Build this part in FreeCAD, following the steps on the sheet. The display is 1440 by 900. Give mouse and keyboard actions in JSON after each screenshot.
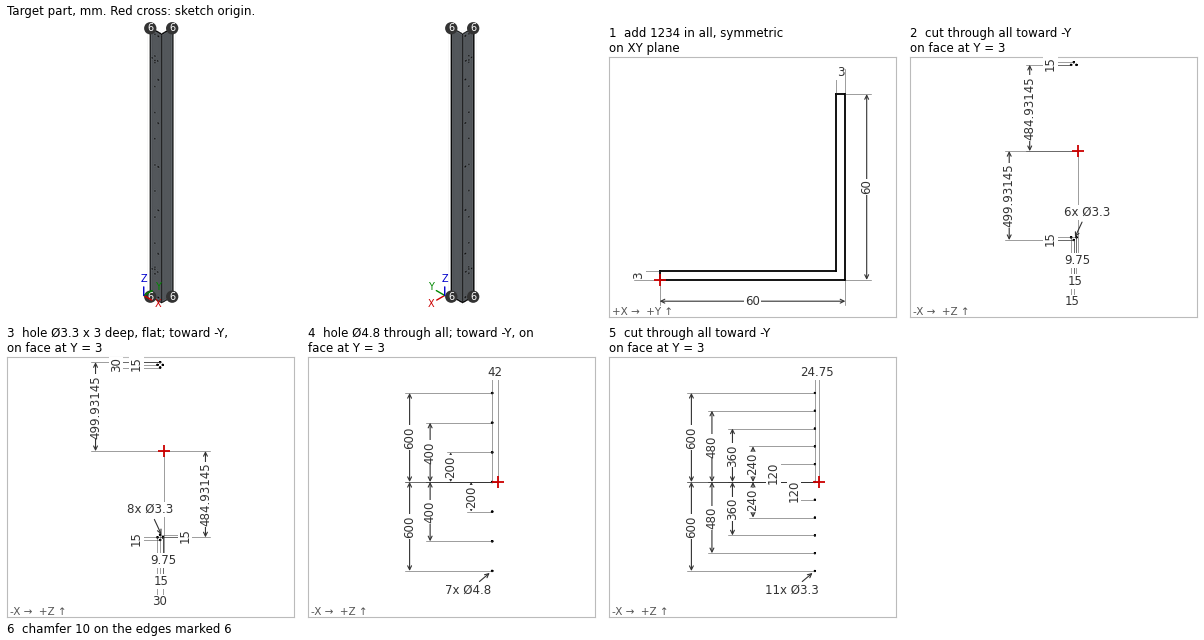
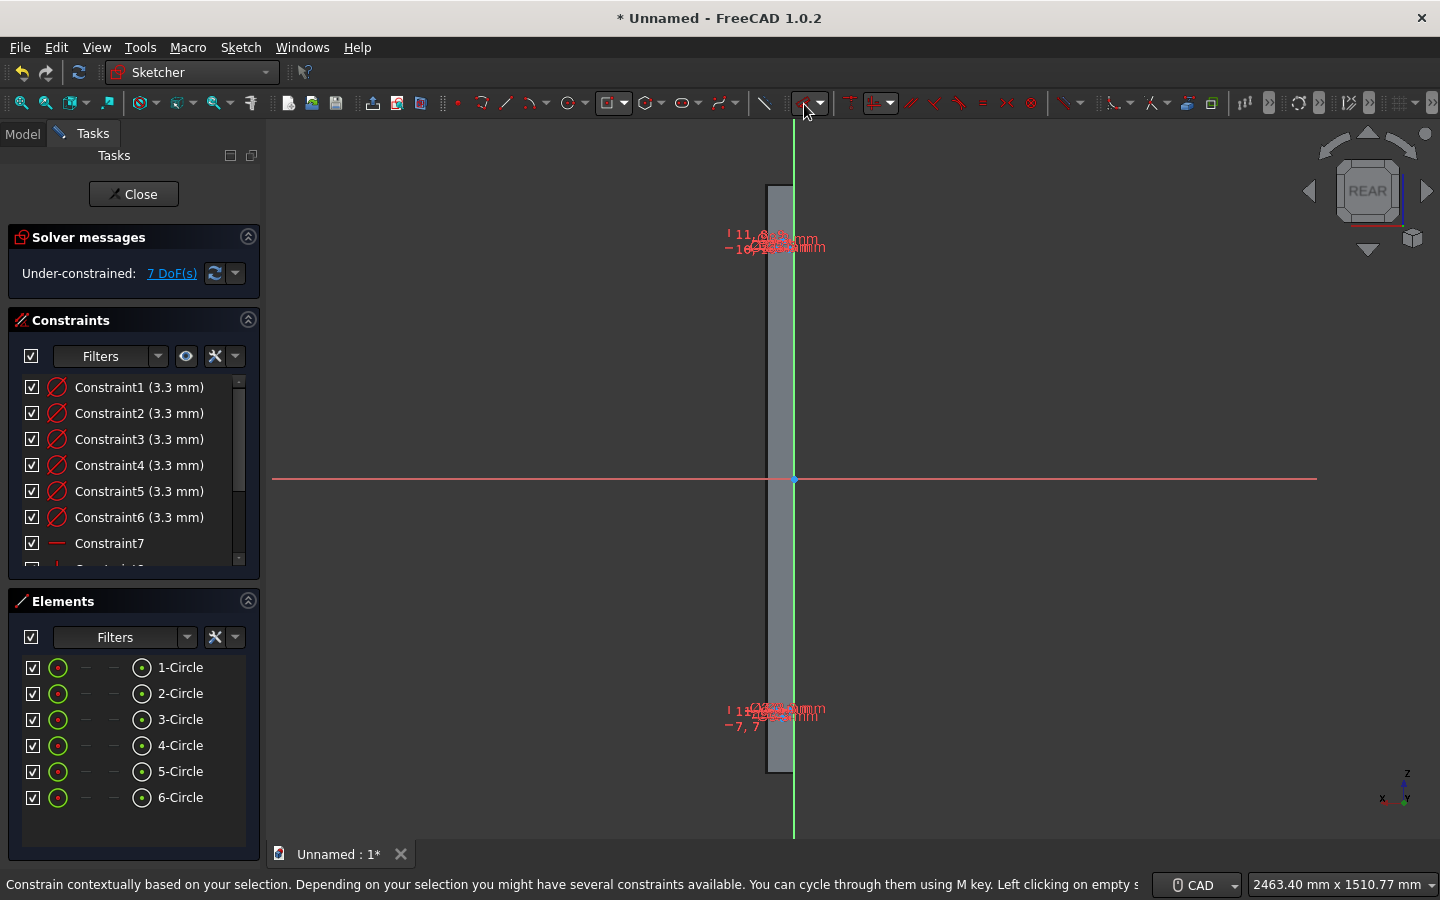
{"action": "scroll", "coordinate": [782, 718], "scroll_direction": "up", "scroll_amount": 9}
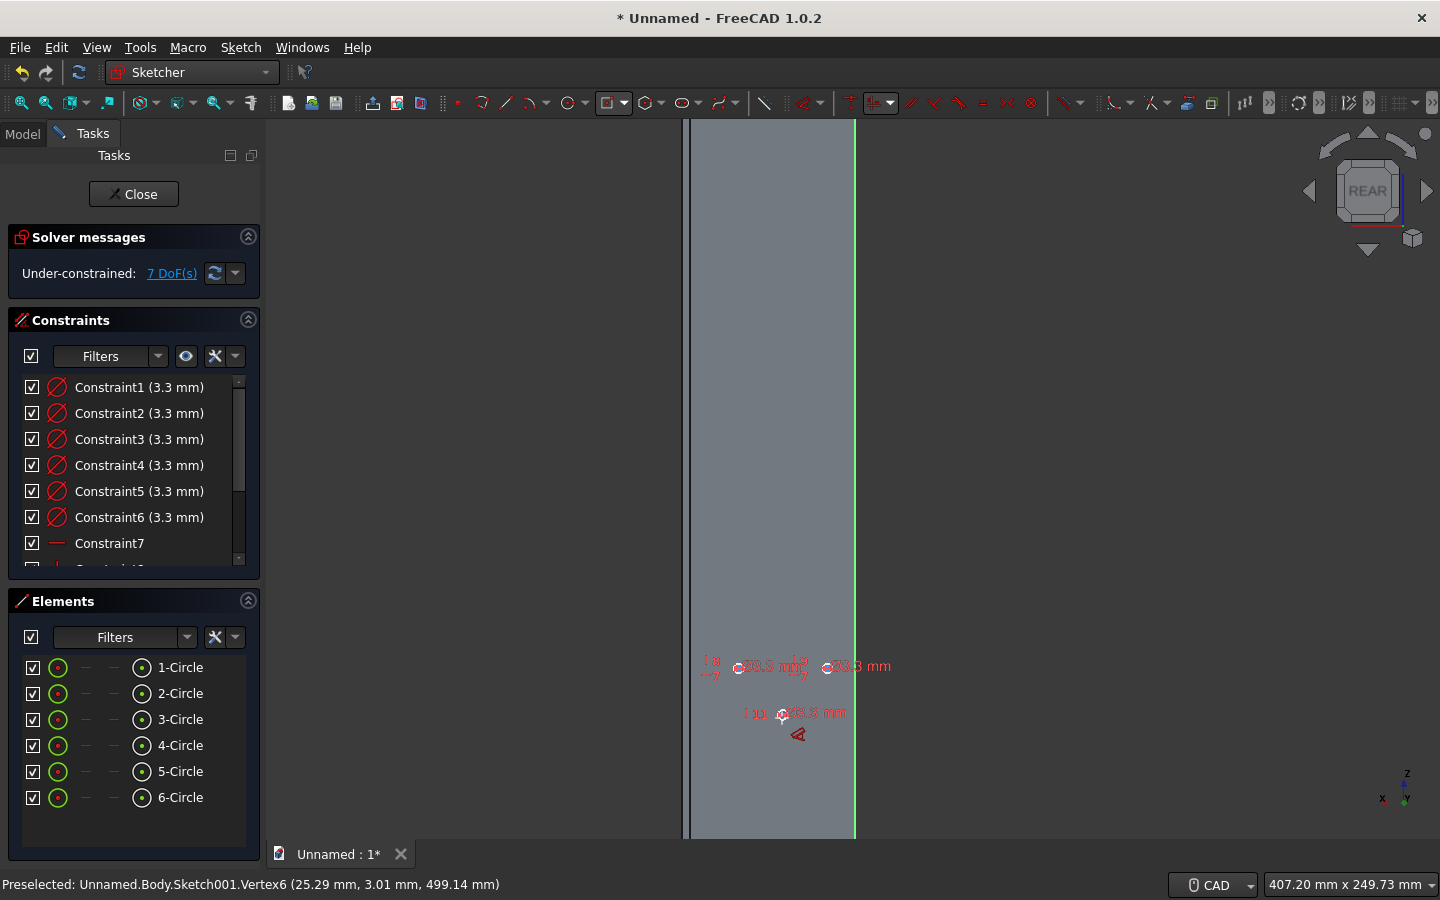
{"action": "left_click", "coordinate": [783, 715]}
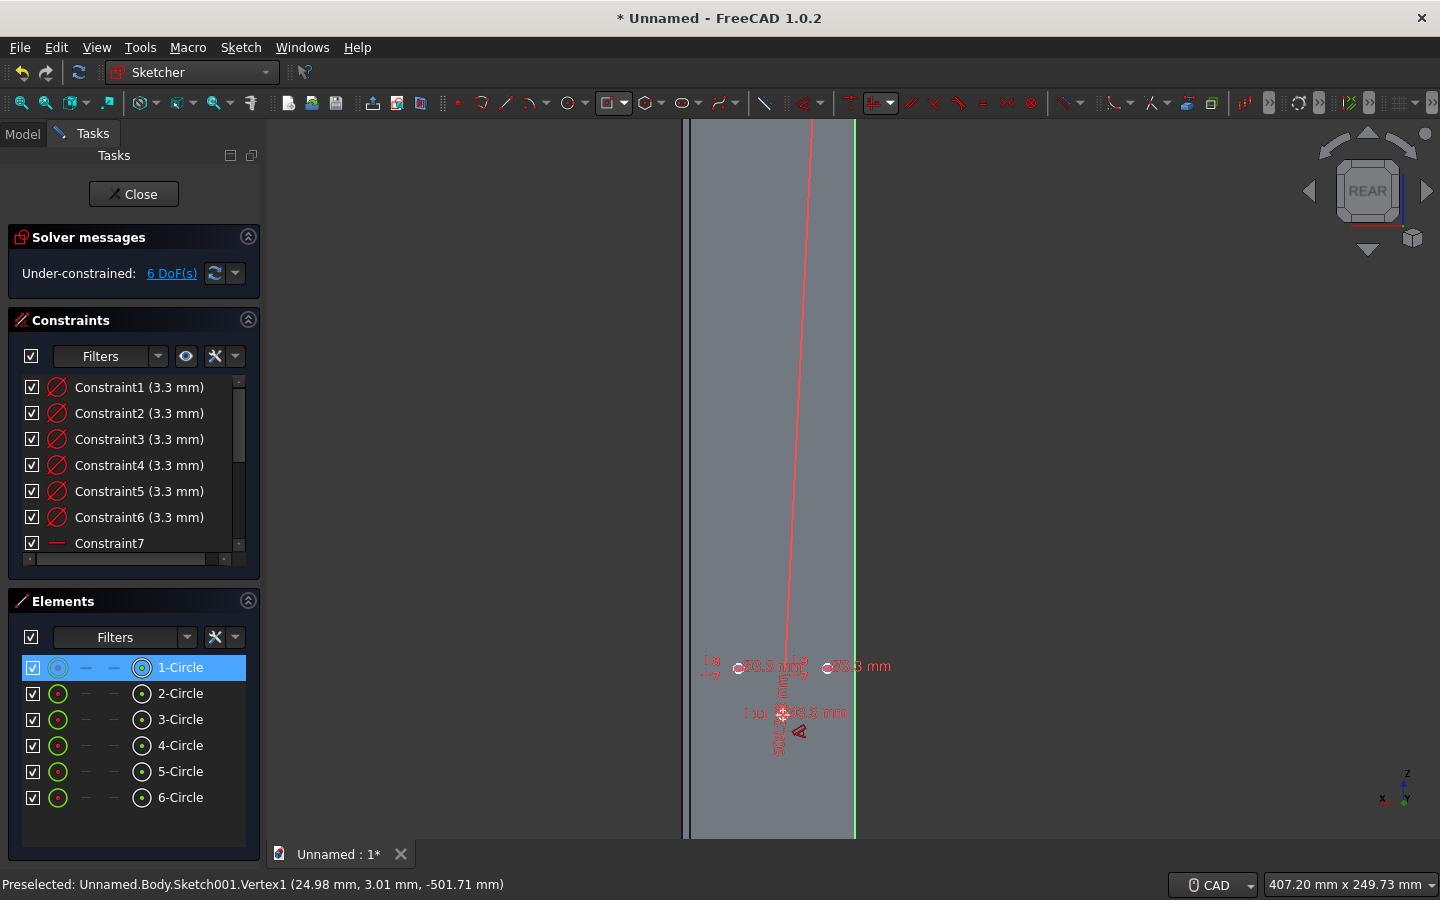
{"action": "left_click", "coordinate": [827, 668]}
{"action": "left_click", "coordinate": [805, 749]}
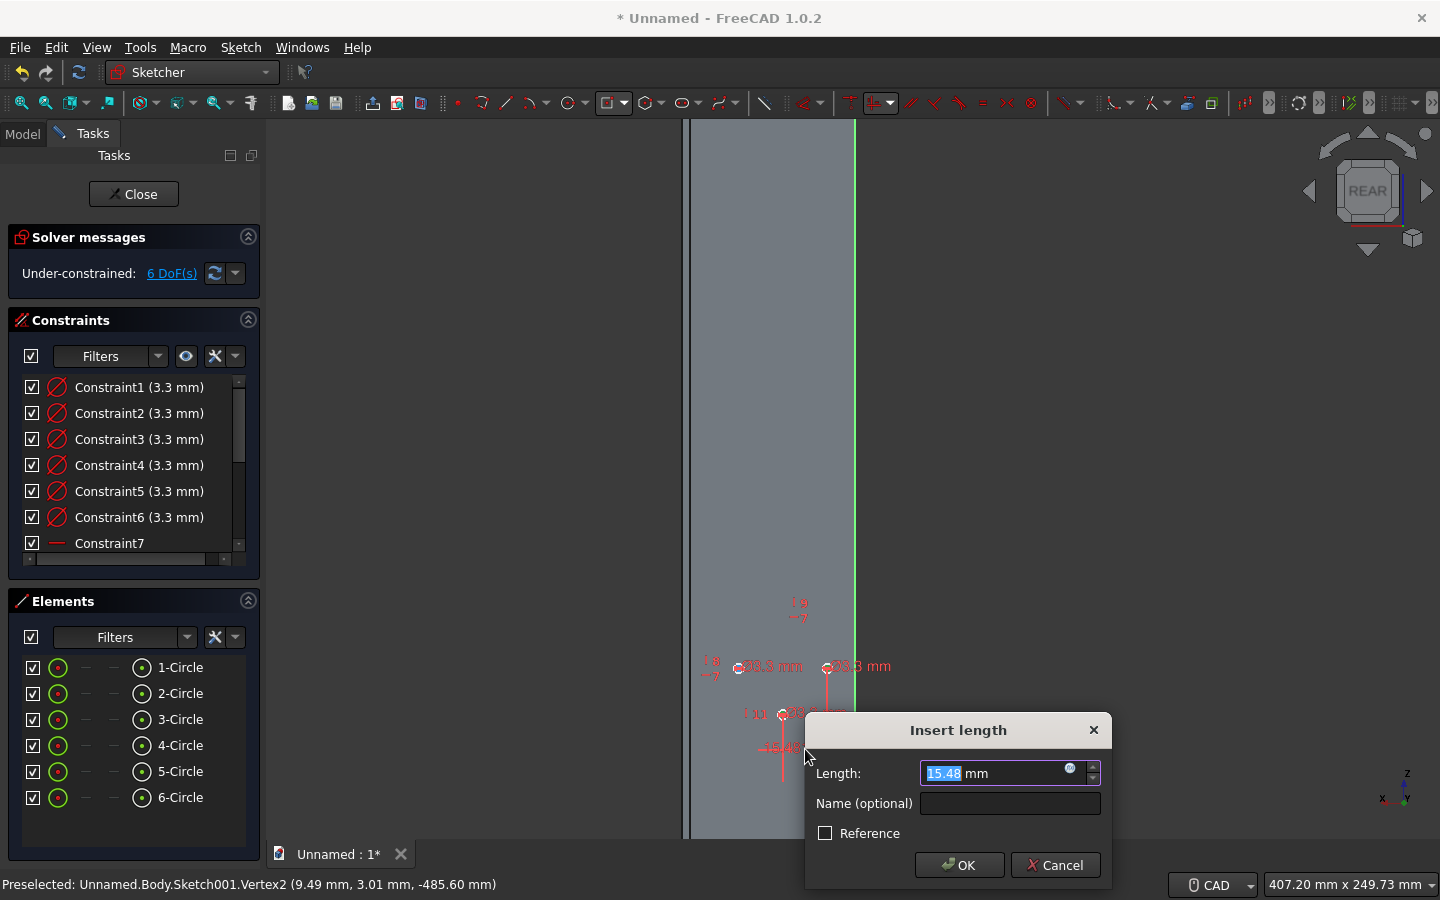
{"action": "type", "text": "15"}
{"action": "key", "text": "Return"}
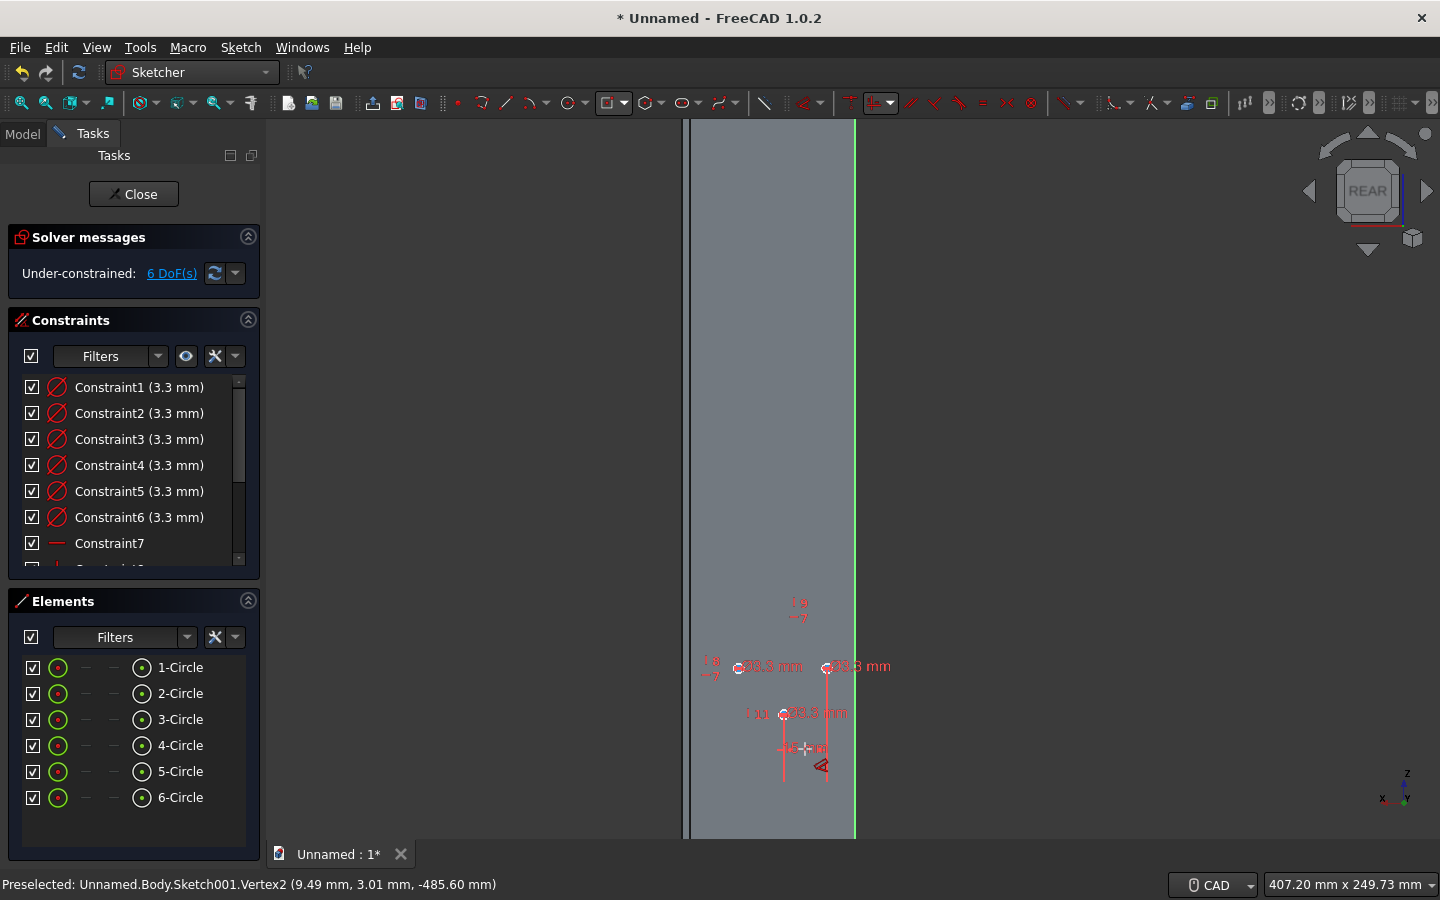
{"action": "left_click", "coordinate": [784, 715]}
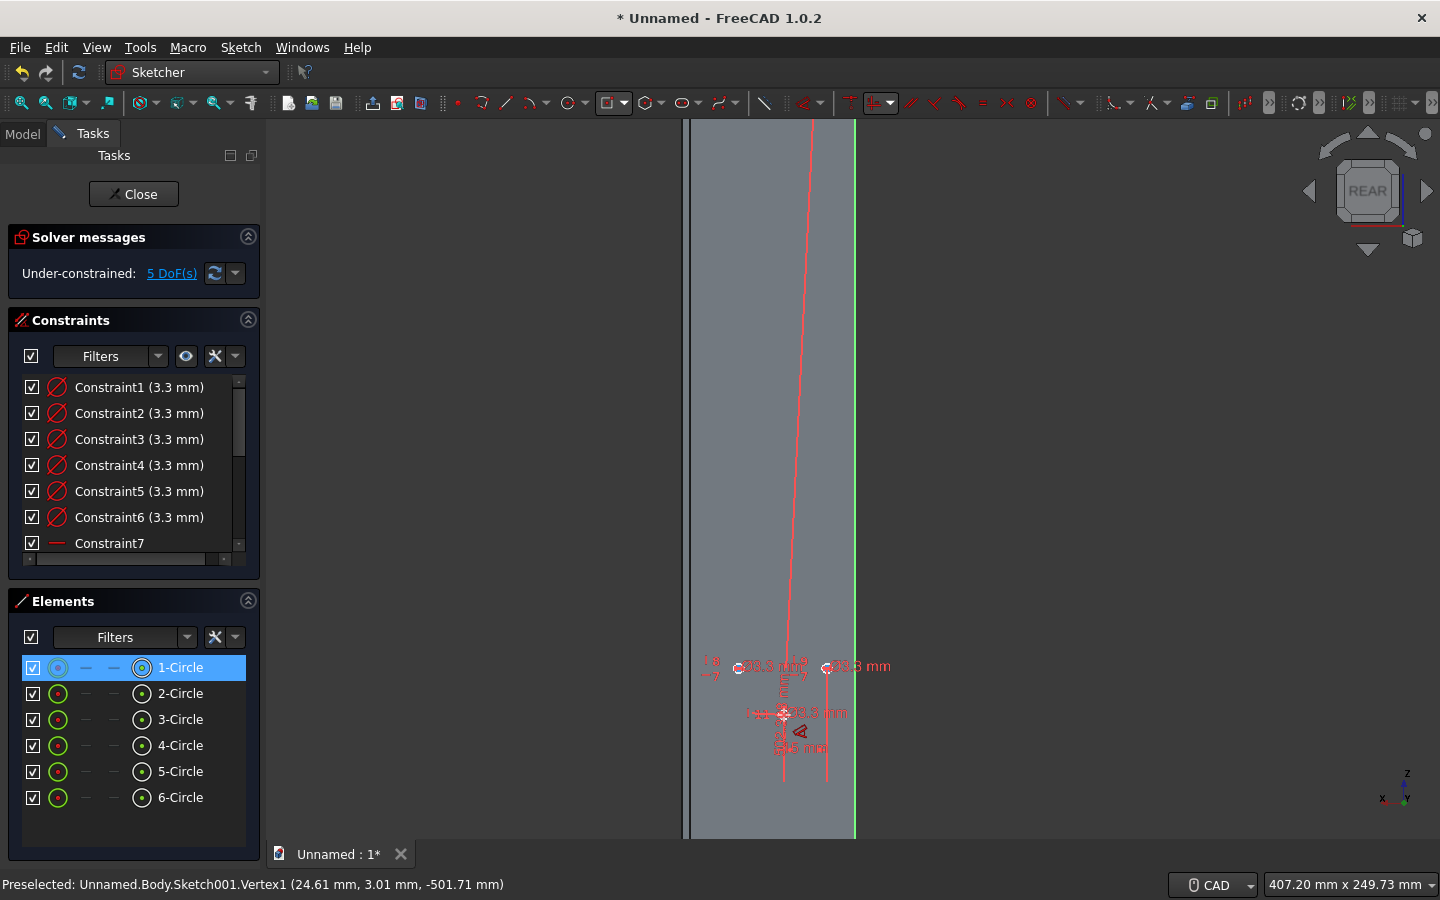
{"action": "left_click", "coordinate": [827, 668]}
{"action": "left_click", "coordinate": [750, 692]}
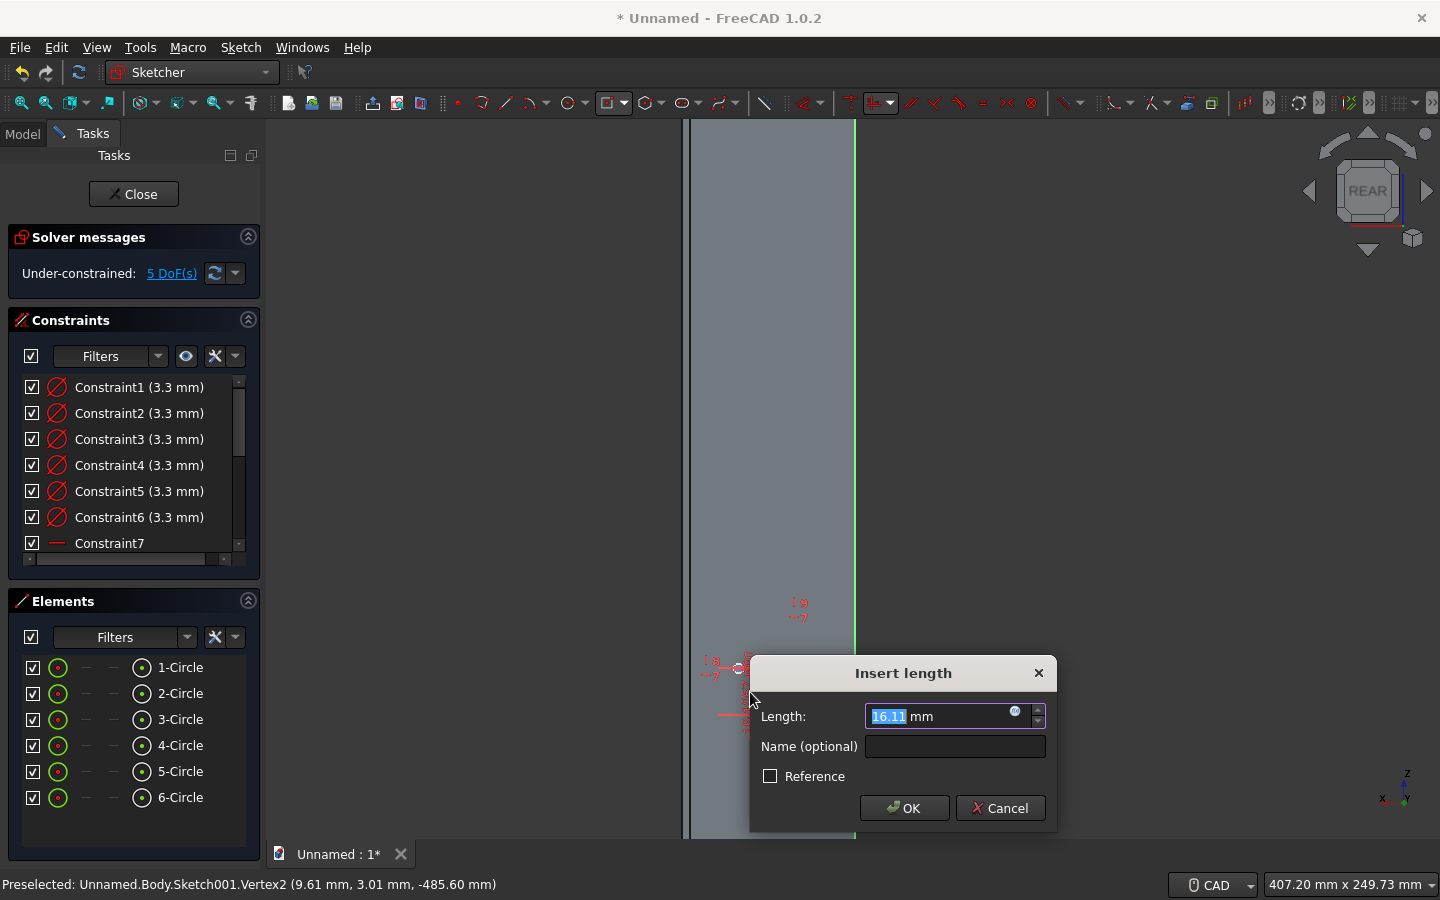
{"action": "type", "text": "15"}
{"action": "key", "text": "Return"}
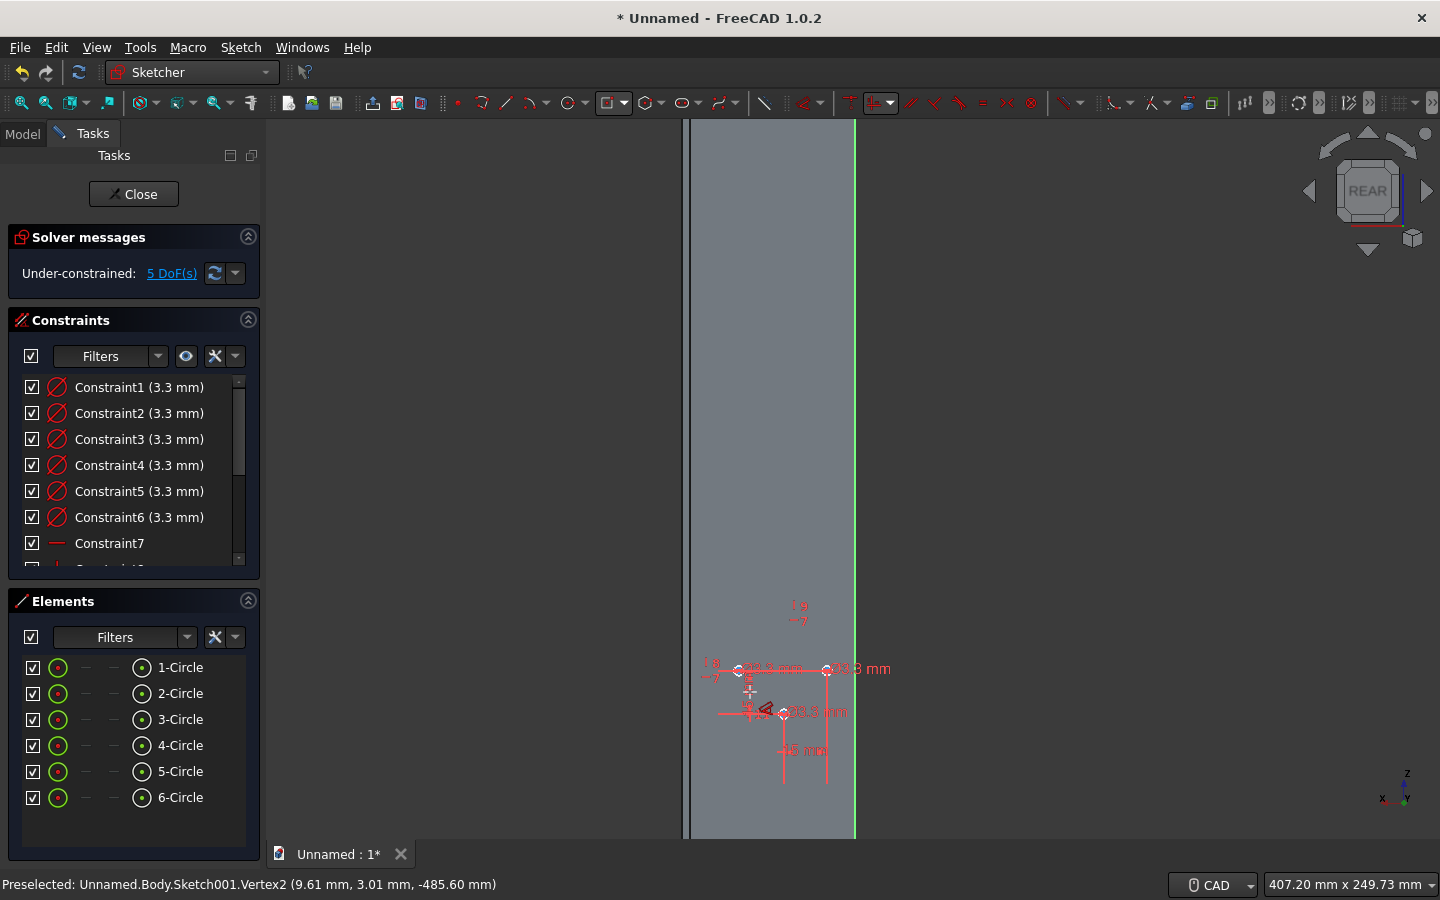
{"action": "left_click", "coordinate": [784, 714]}